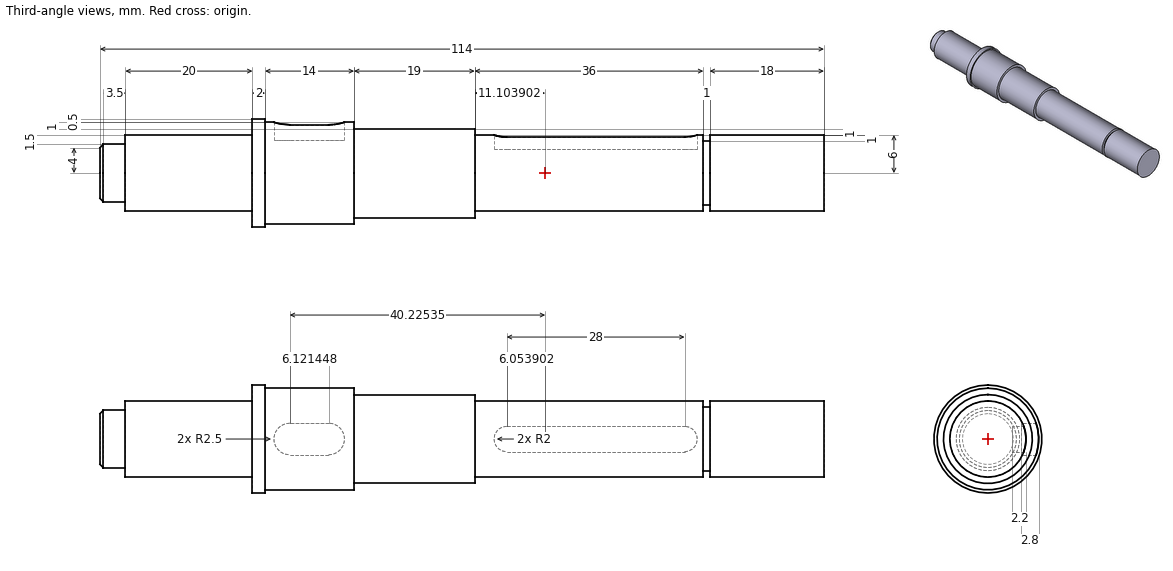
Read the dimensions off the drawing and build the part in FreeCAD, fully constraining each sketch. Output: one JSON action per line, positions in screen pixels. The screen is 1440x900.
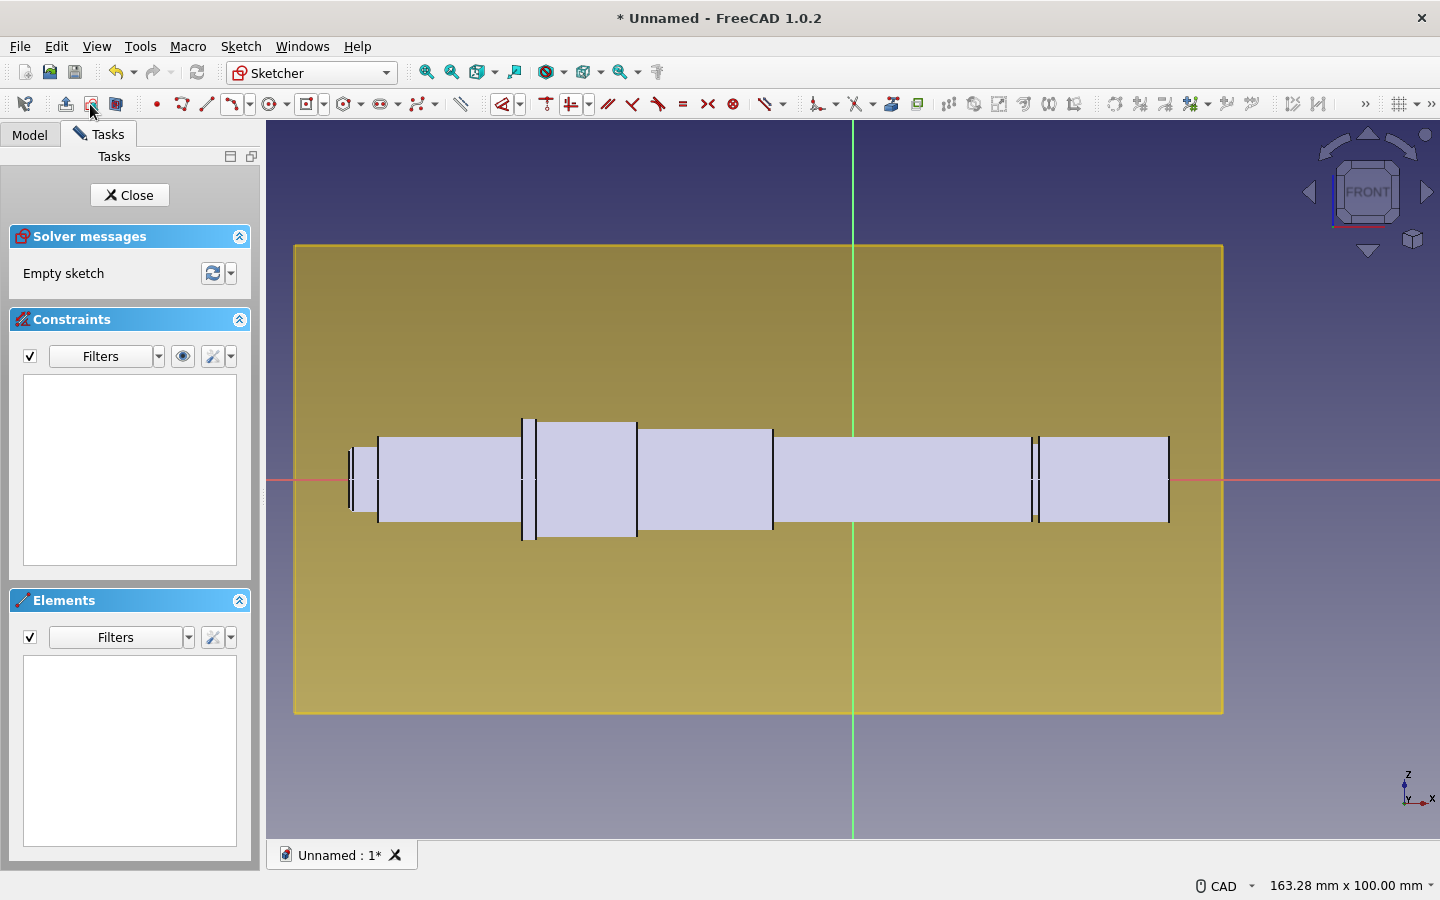
{"action": "left_click", "coordinate": [116, 104]}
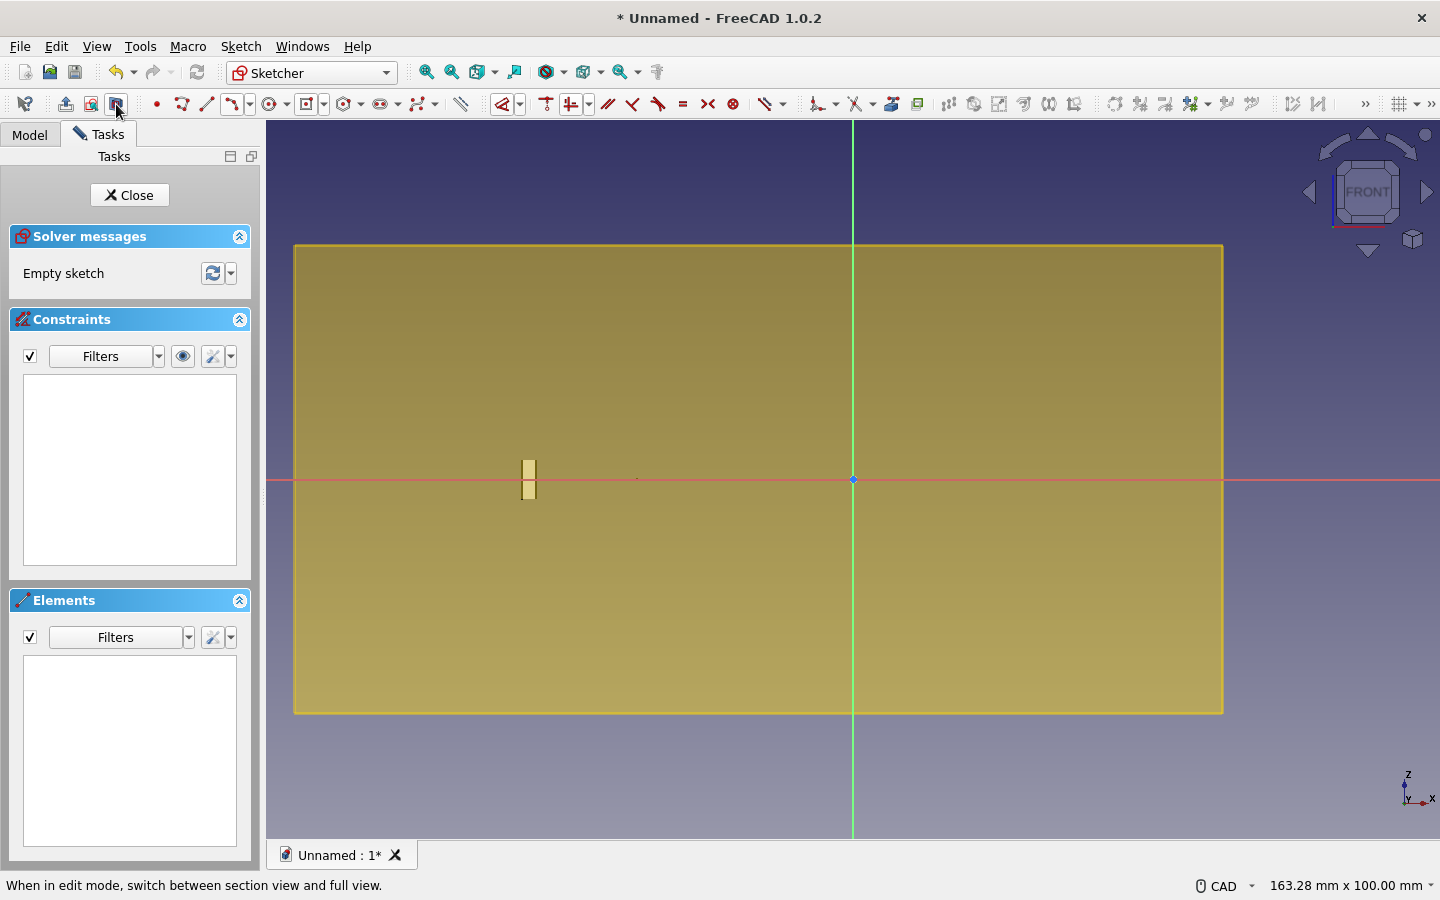
{"action": "scroll", "coordinate": [561, 479], "scroll_direction": "up", "scroll_amount": 11}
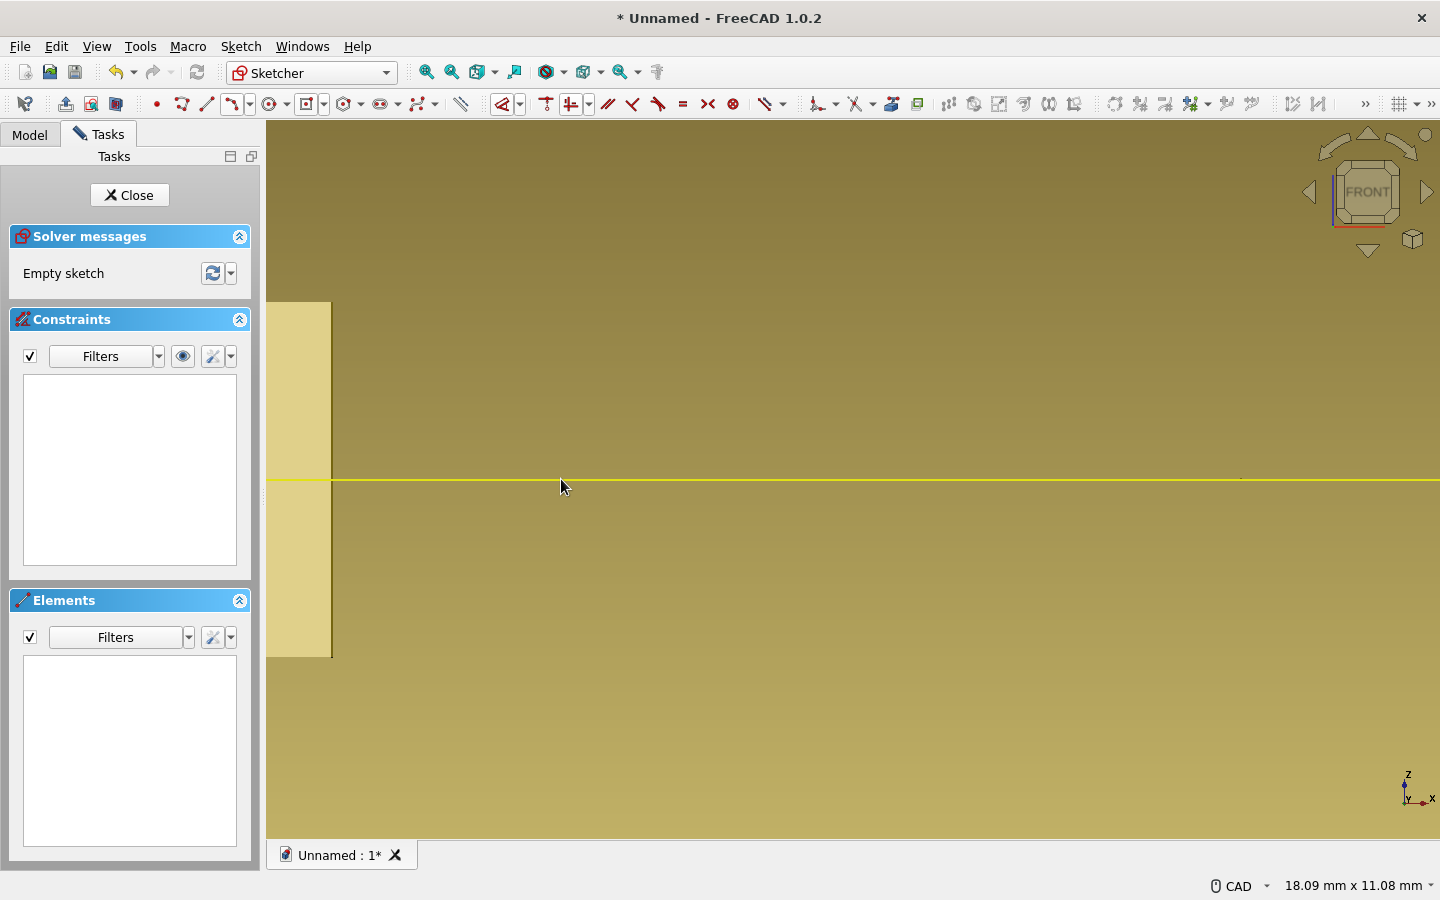
{"action": "left_click", "coordinate": [380, 104]}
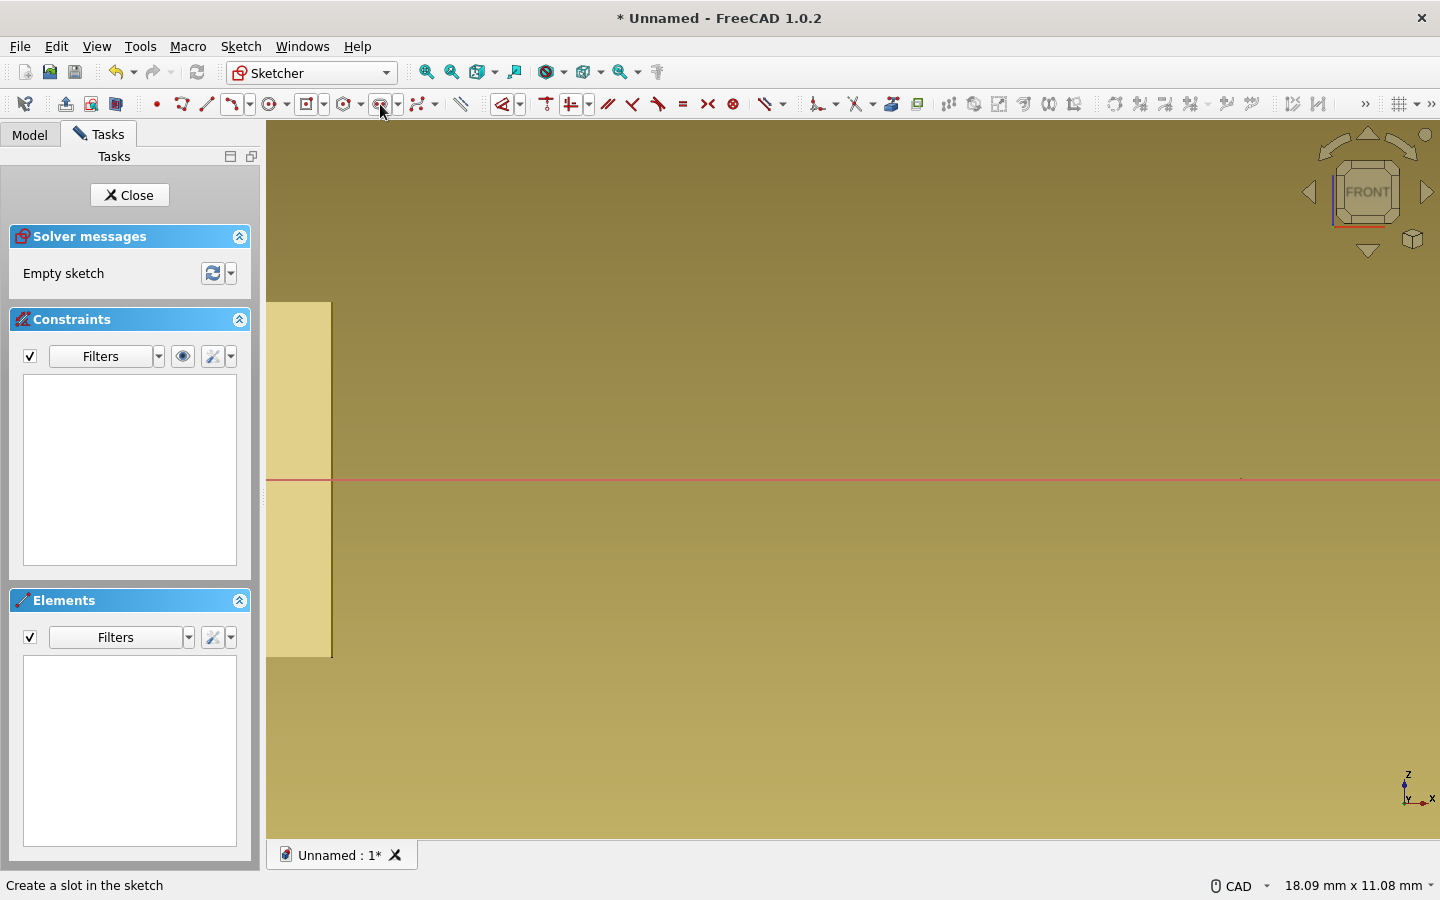
{"action": "left_click", "coordinate": [584, 480]}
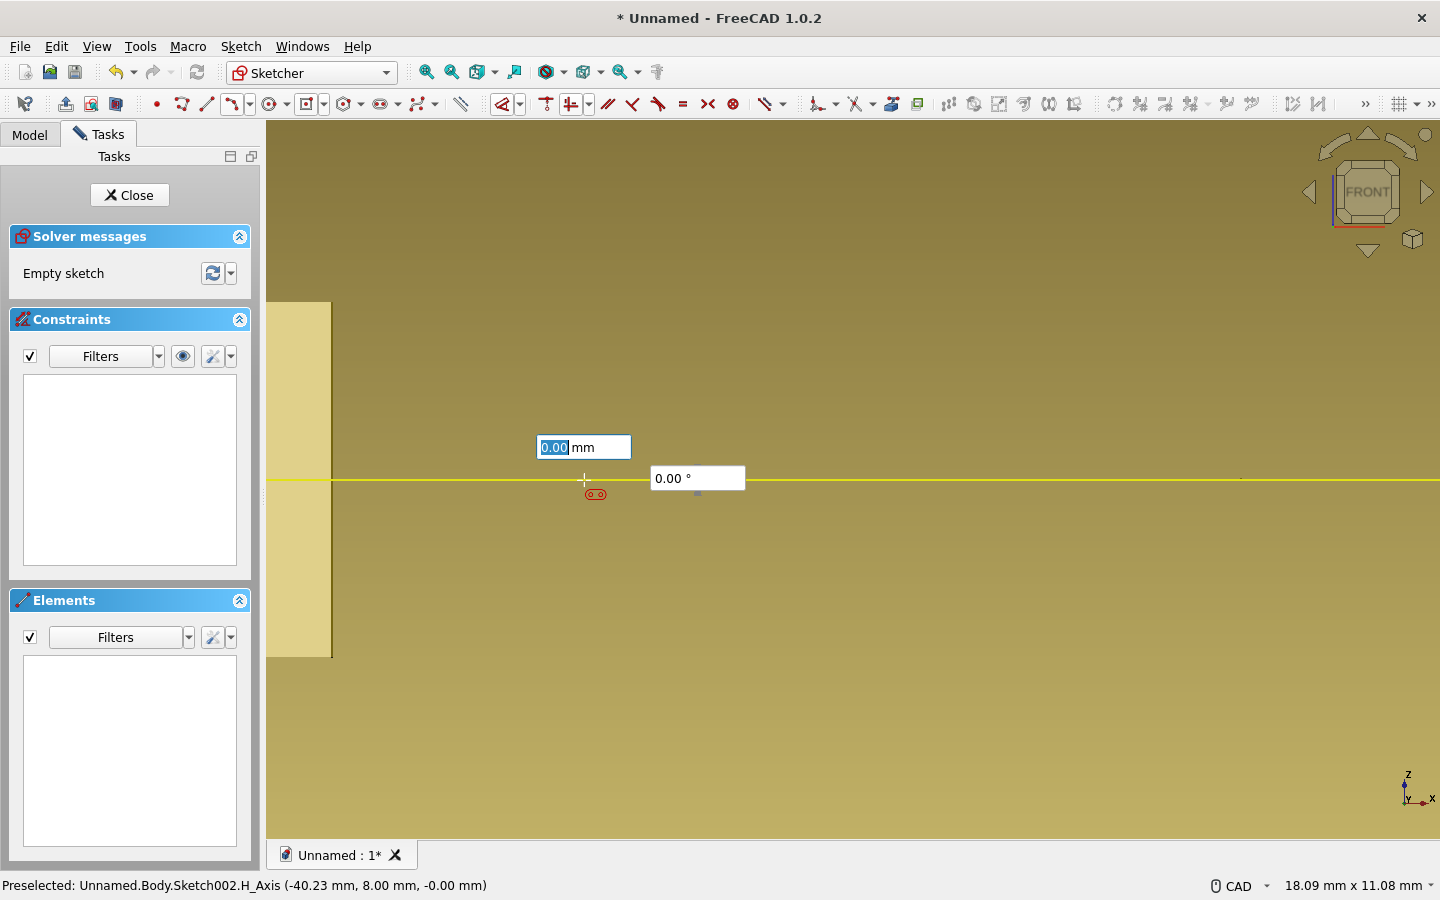
{"action": "left_click", "coordinate": [981, 471]}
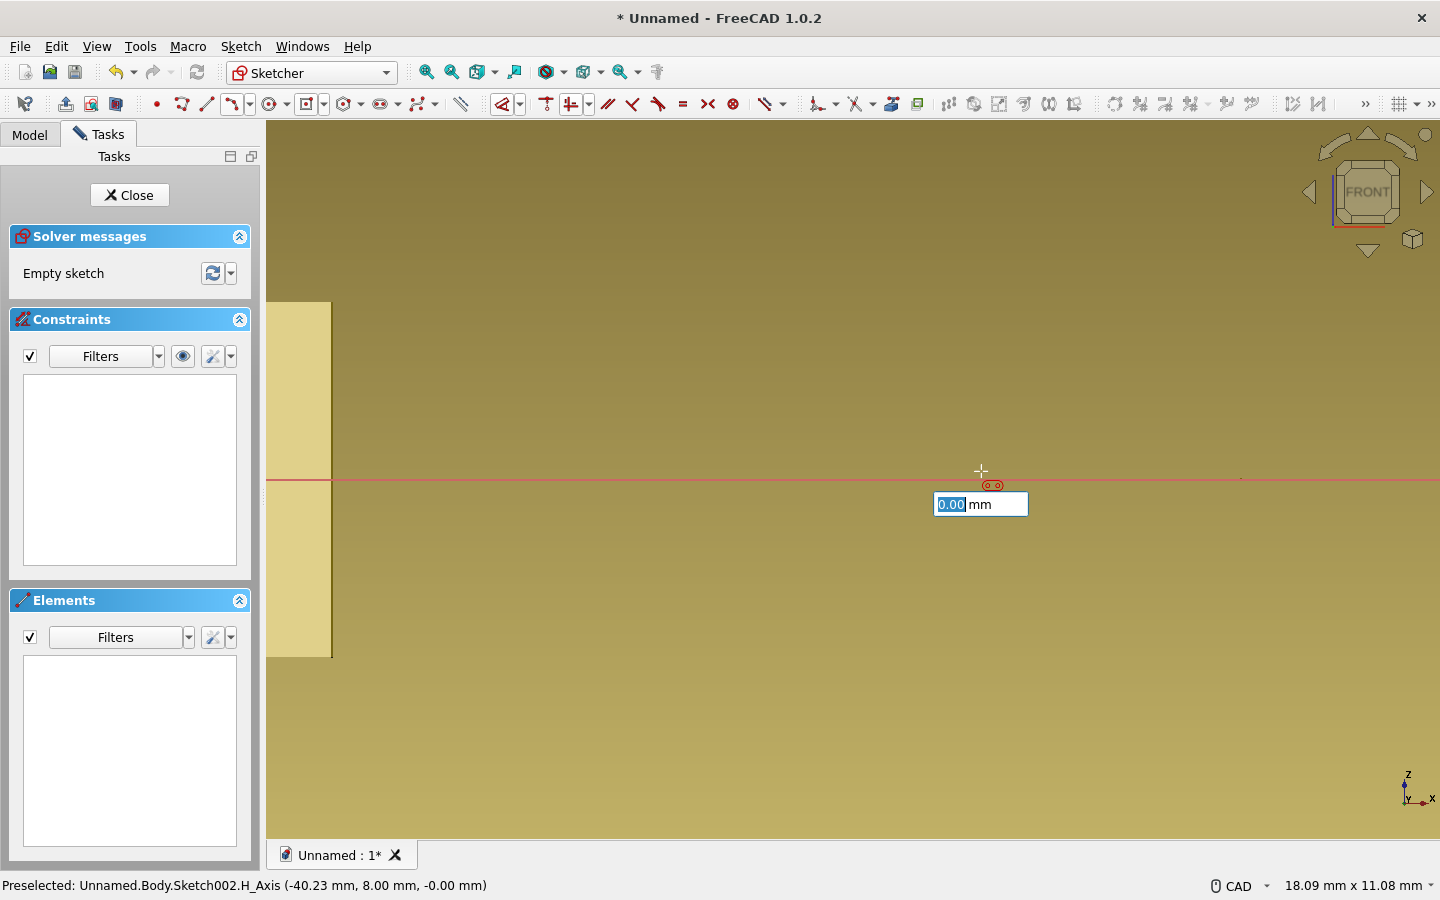
{"action": "left_click", "coordinate": [783, 642]}
{"action": "key", "text": "Escape"}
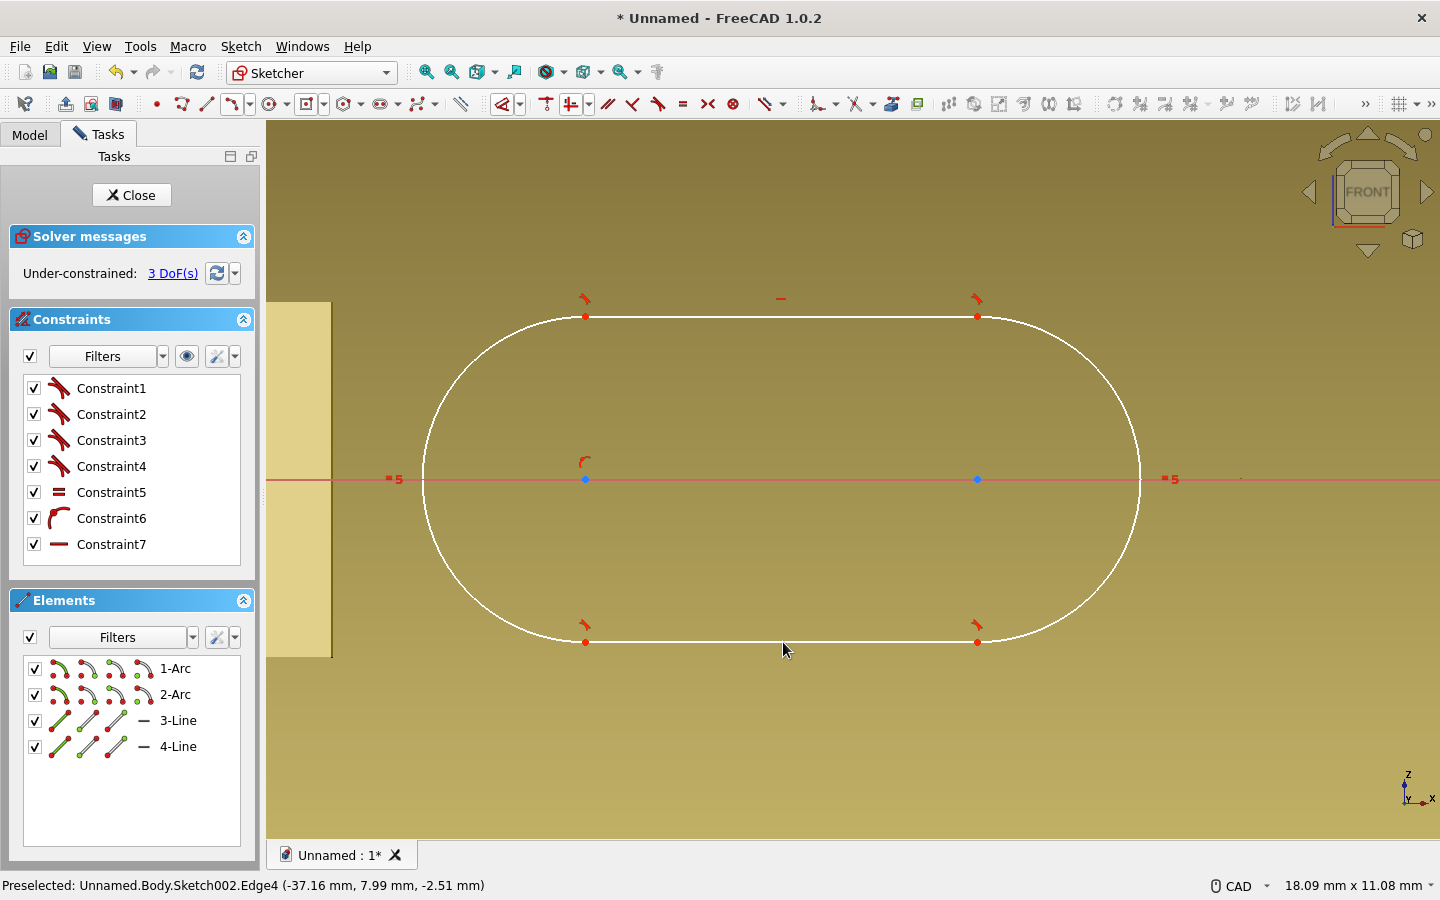
{"action": "left_click", "coordinate": [454, 384]}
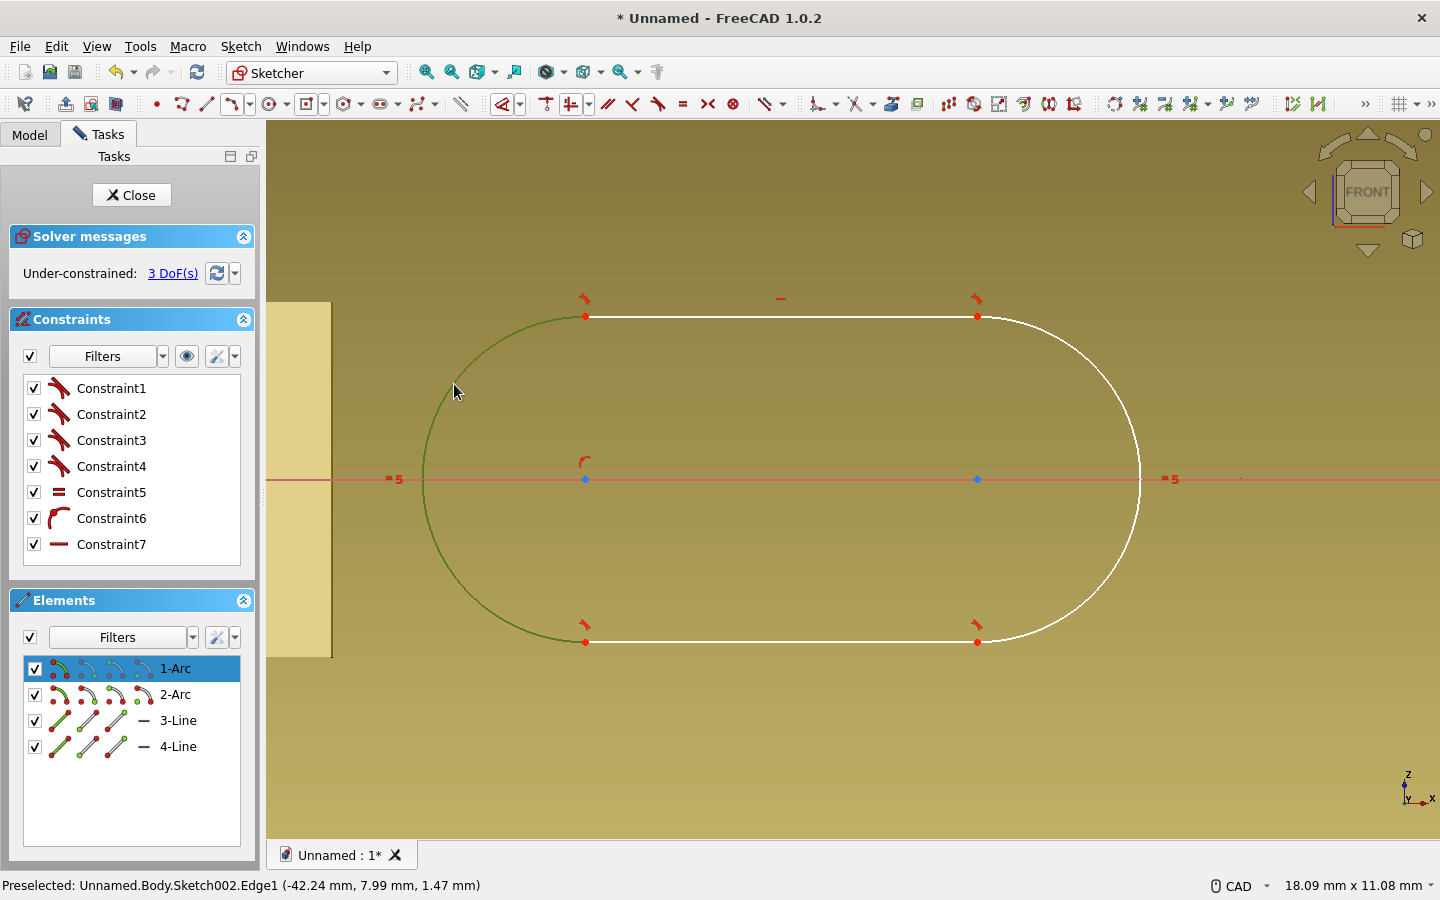
{"action": "left_click", "coordinate": [520, 104]}